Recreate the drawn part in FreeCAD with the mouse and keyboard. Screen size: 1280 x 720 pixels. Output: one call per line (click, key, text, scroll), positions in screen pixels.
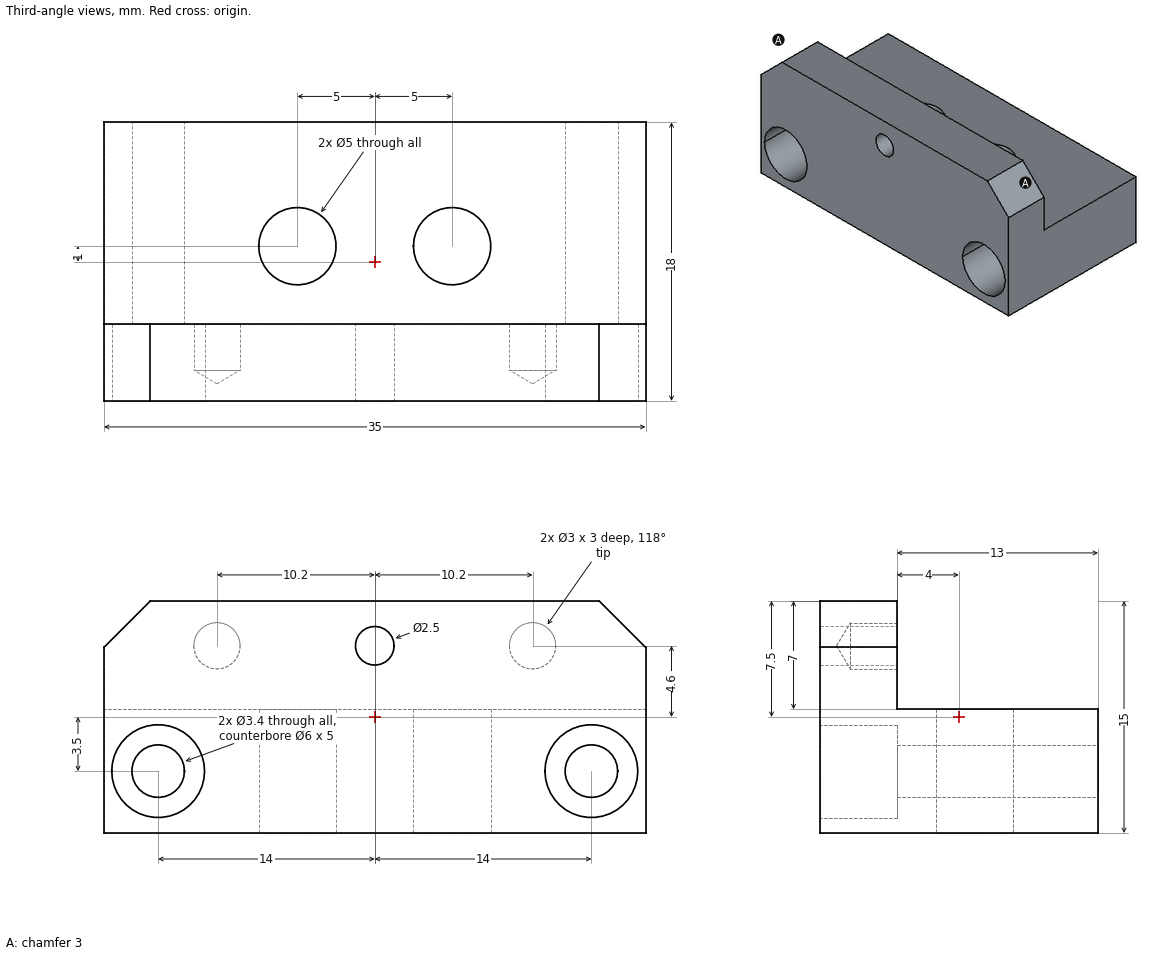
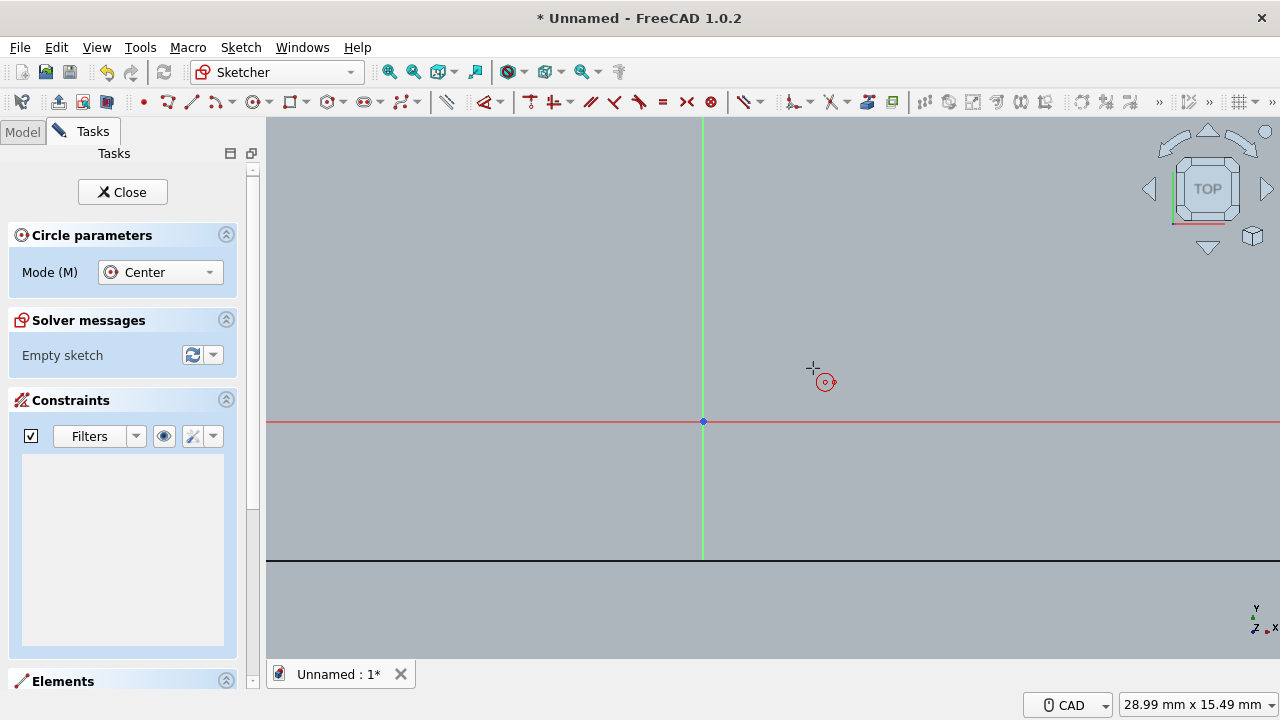
click(528, 387)
click(590, 325)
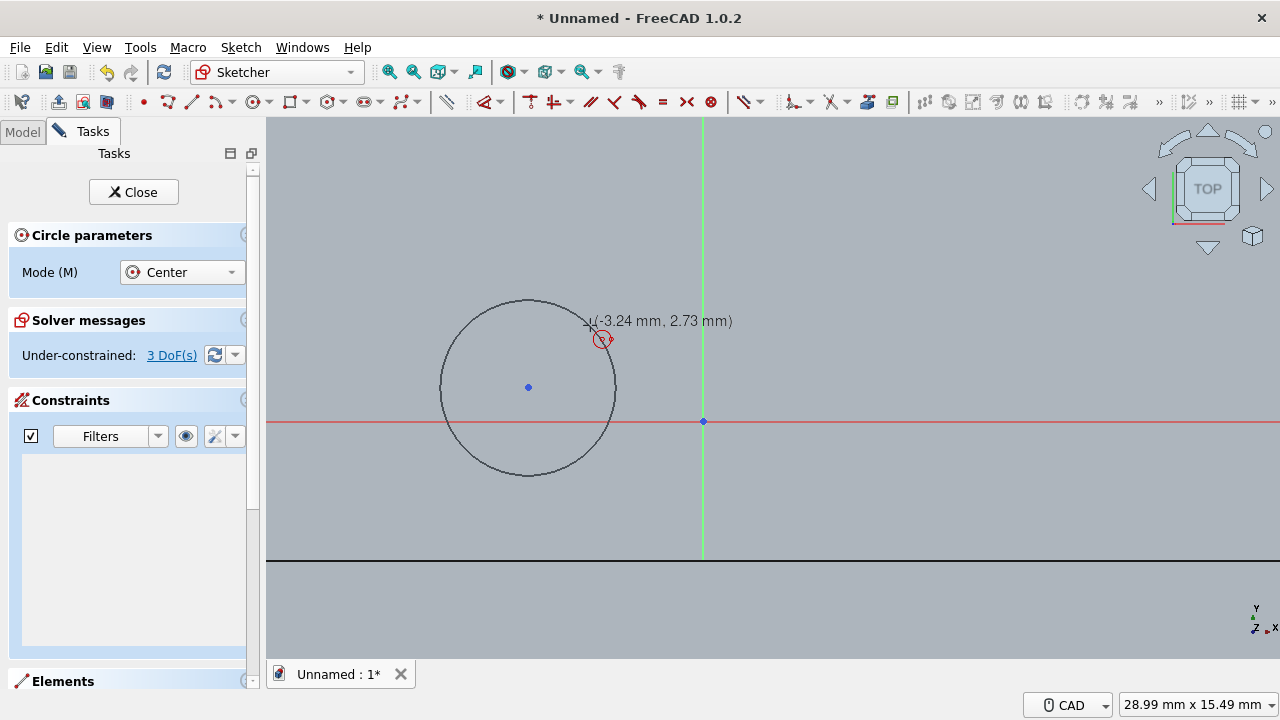
click(878, 387)
click(940, 325)
key(Escape)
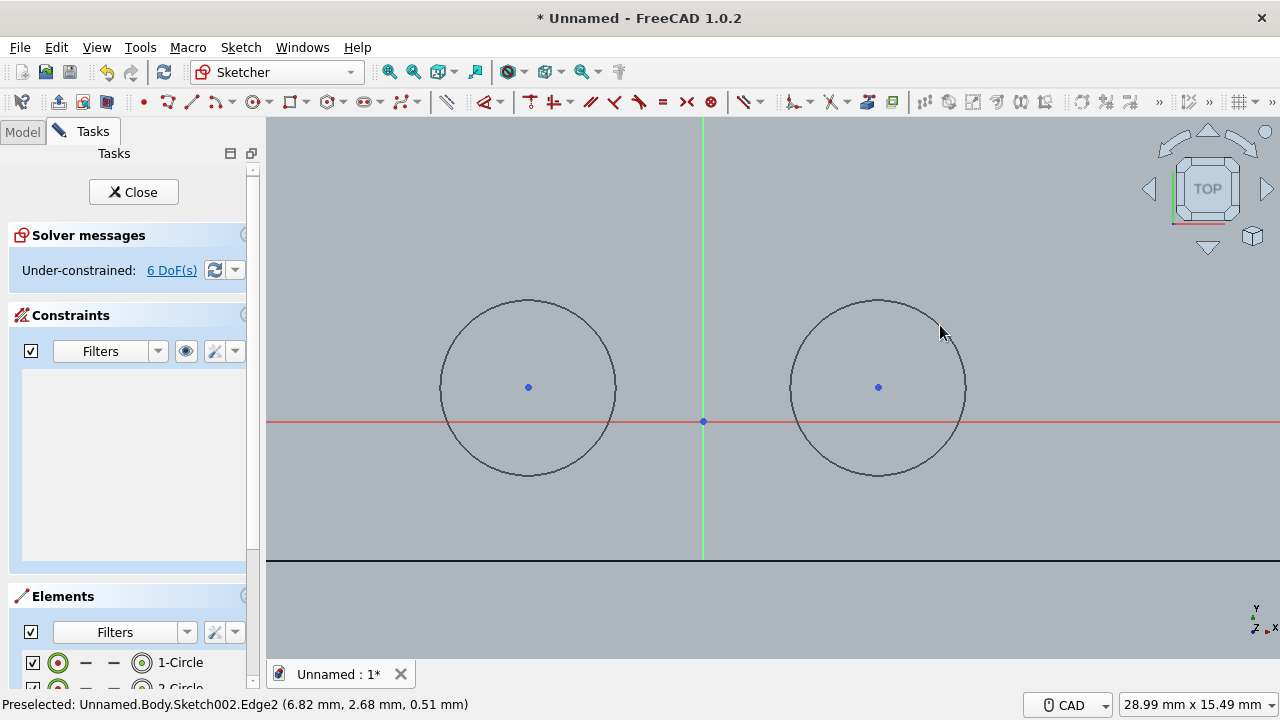
click(590, 326)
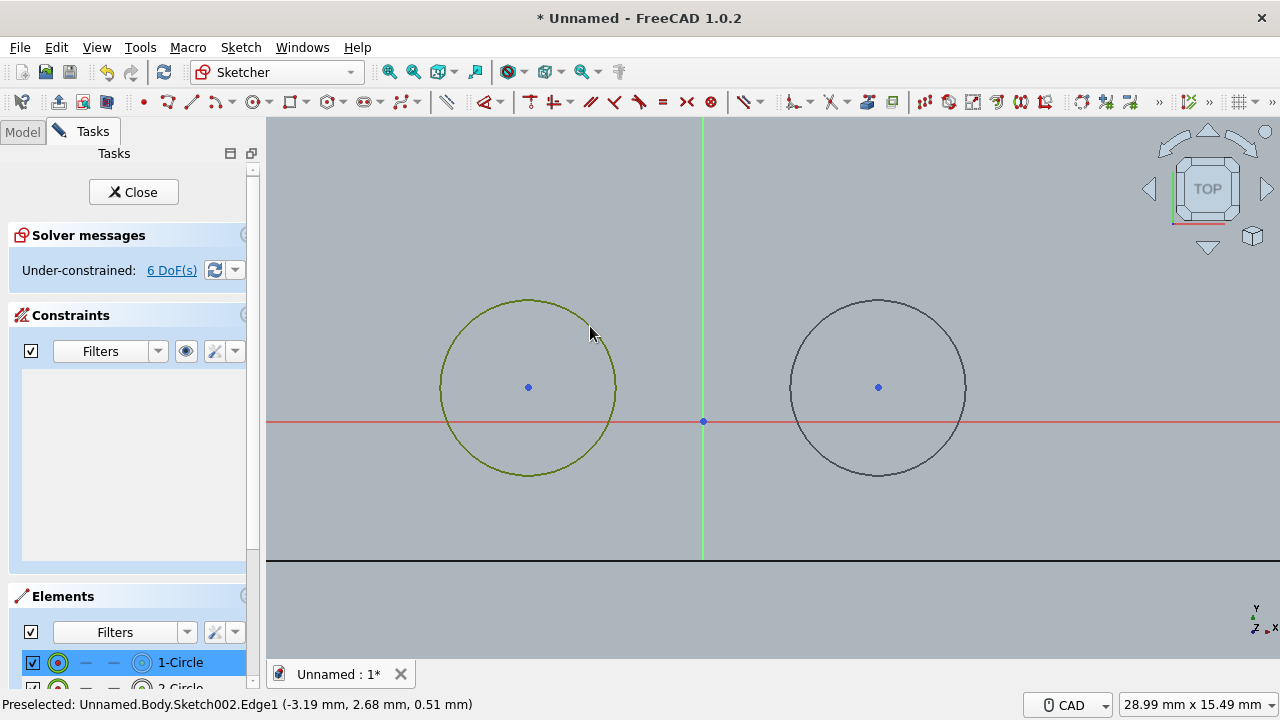
click(940, 326)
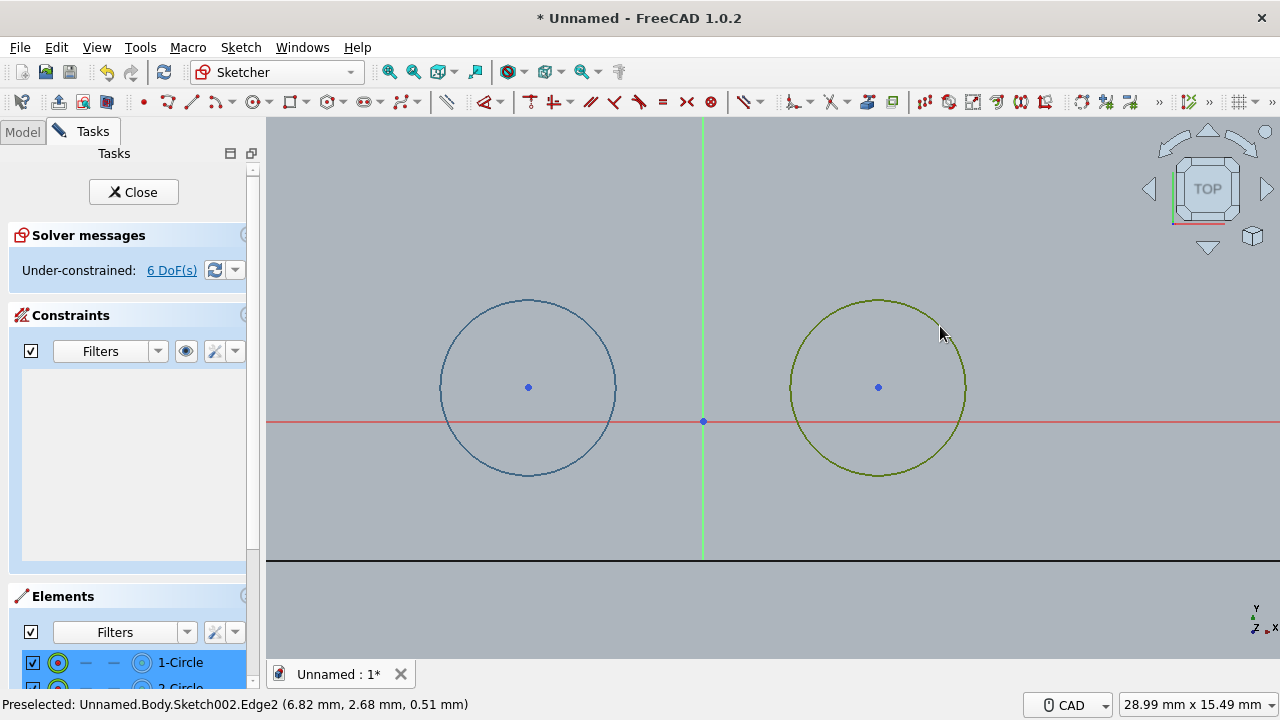
key(e)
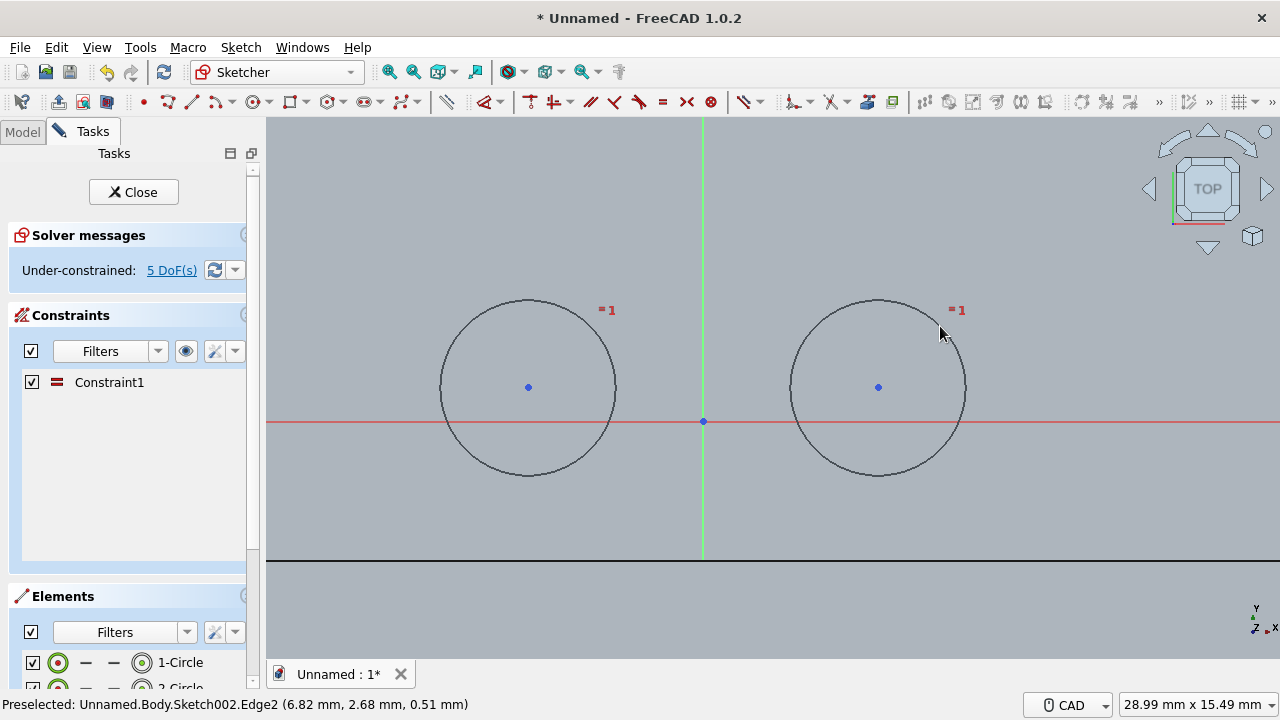
click(528, 388)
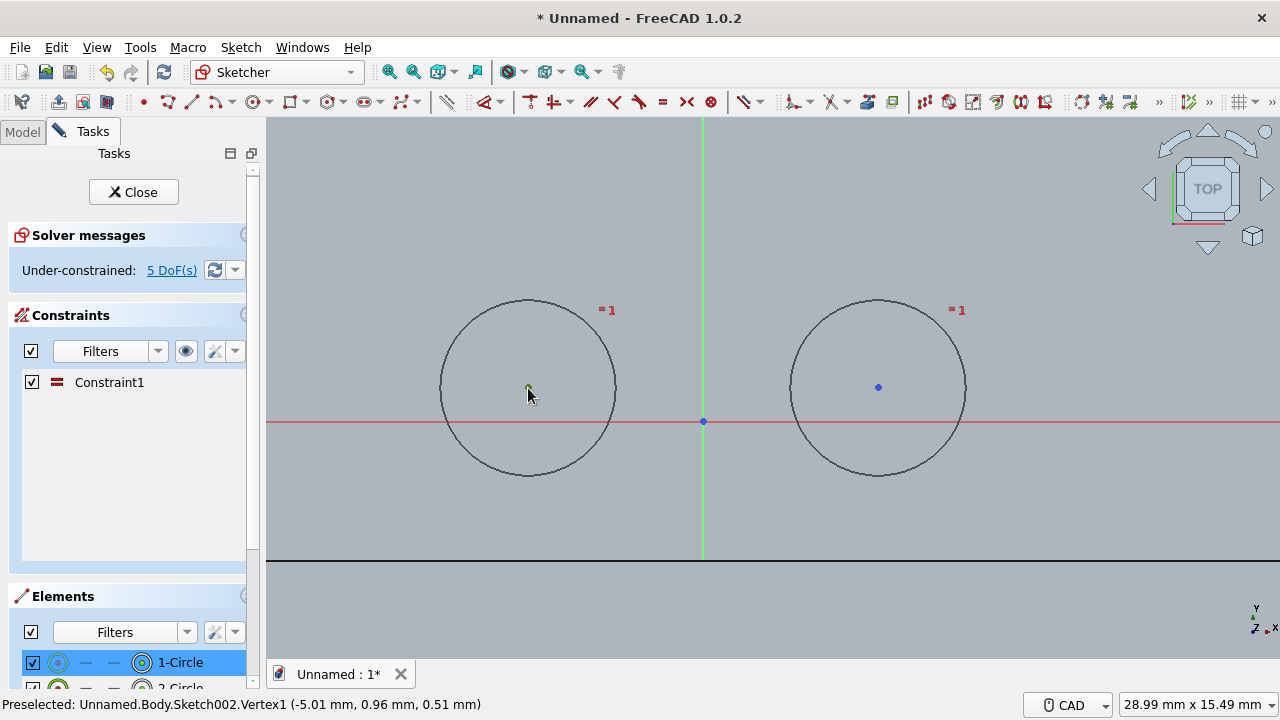
click(878, 388)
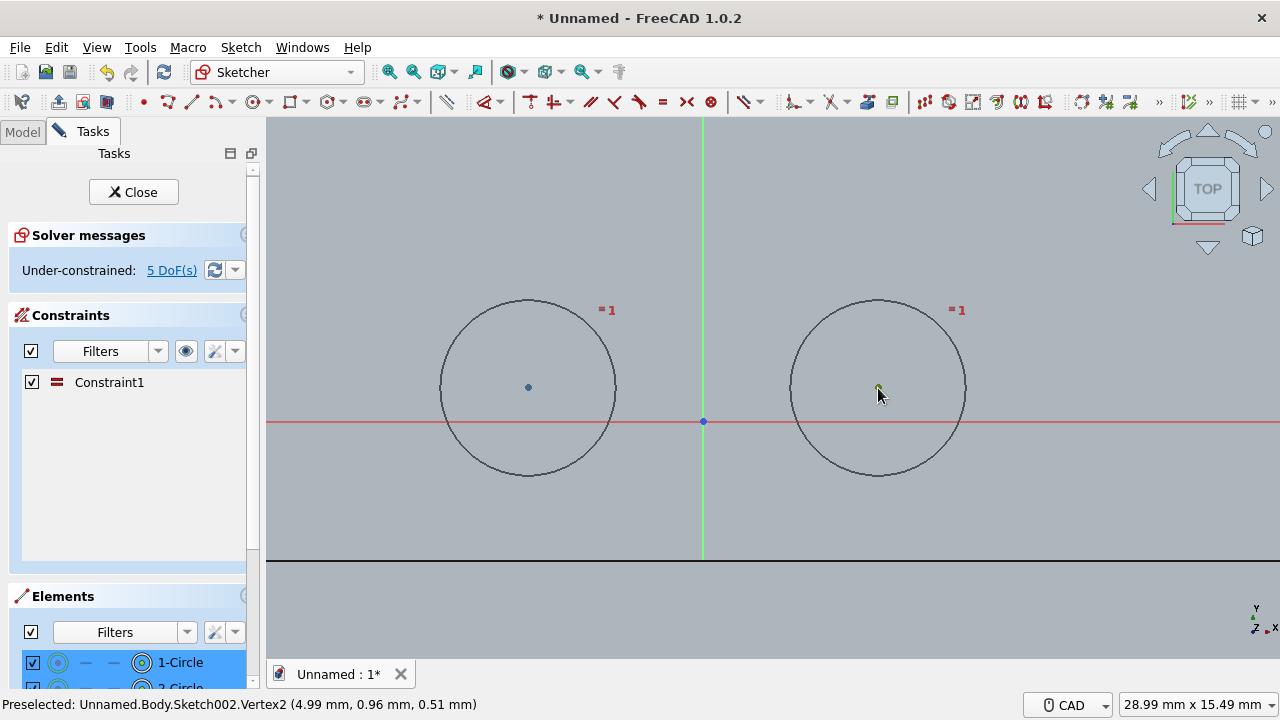
key(h)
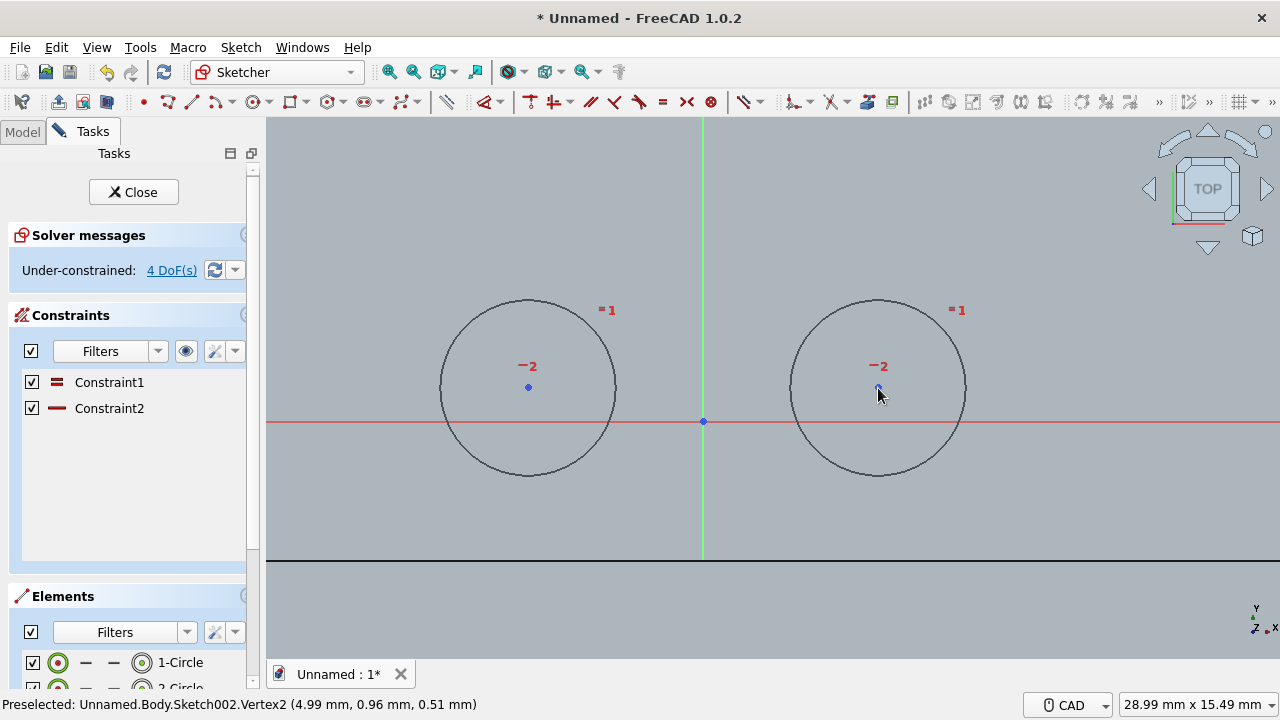
key(d)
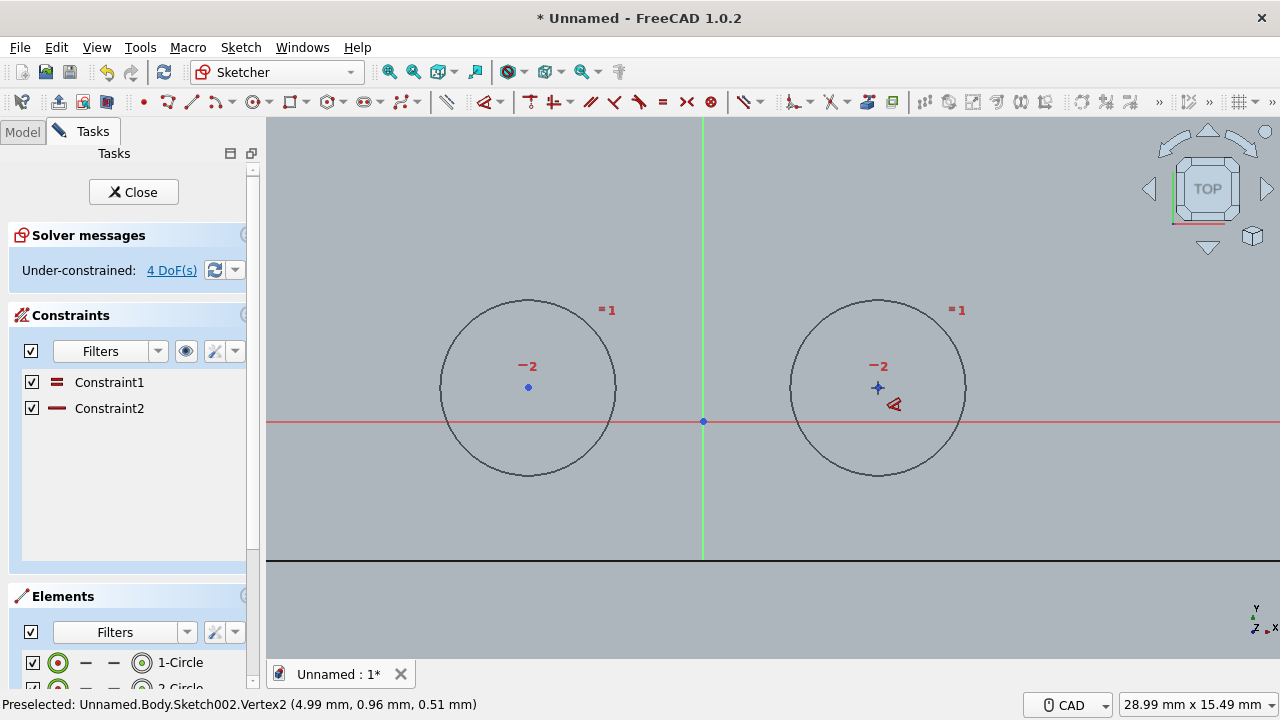
click(590, 326)
click(613, 303)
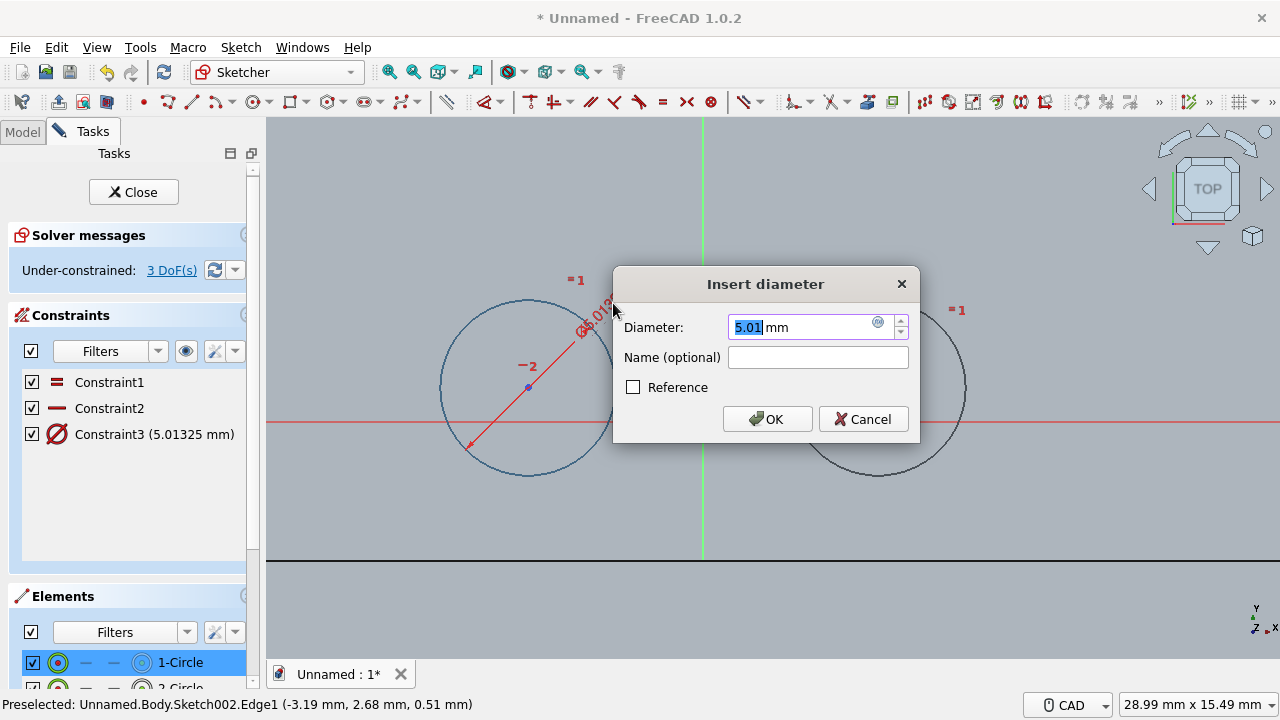
text(5)
key(Return)